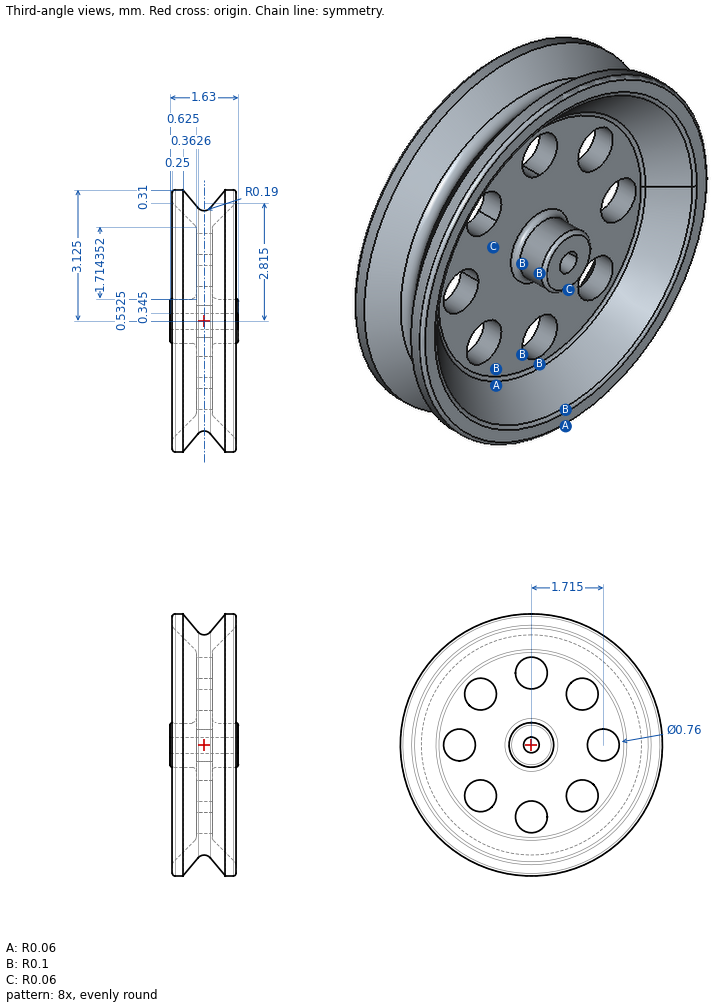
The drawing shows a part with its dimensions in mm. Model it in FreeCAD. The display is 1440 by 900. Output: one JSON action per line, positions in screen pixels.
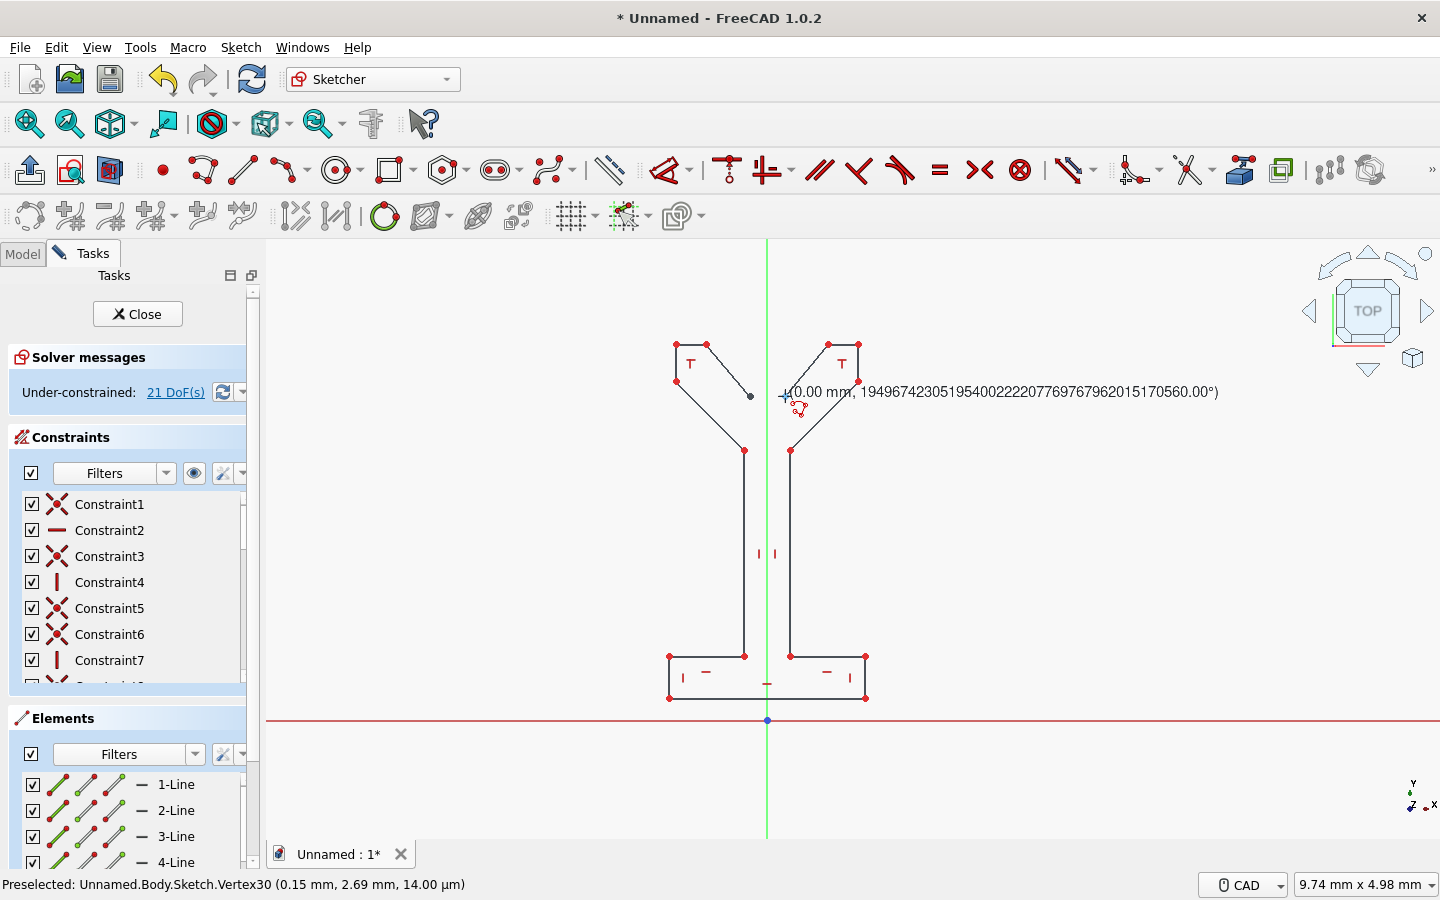
{"action": "left_click", "coordinate": [284, 170]}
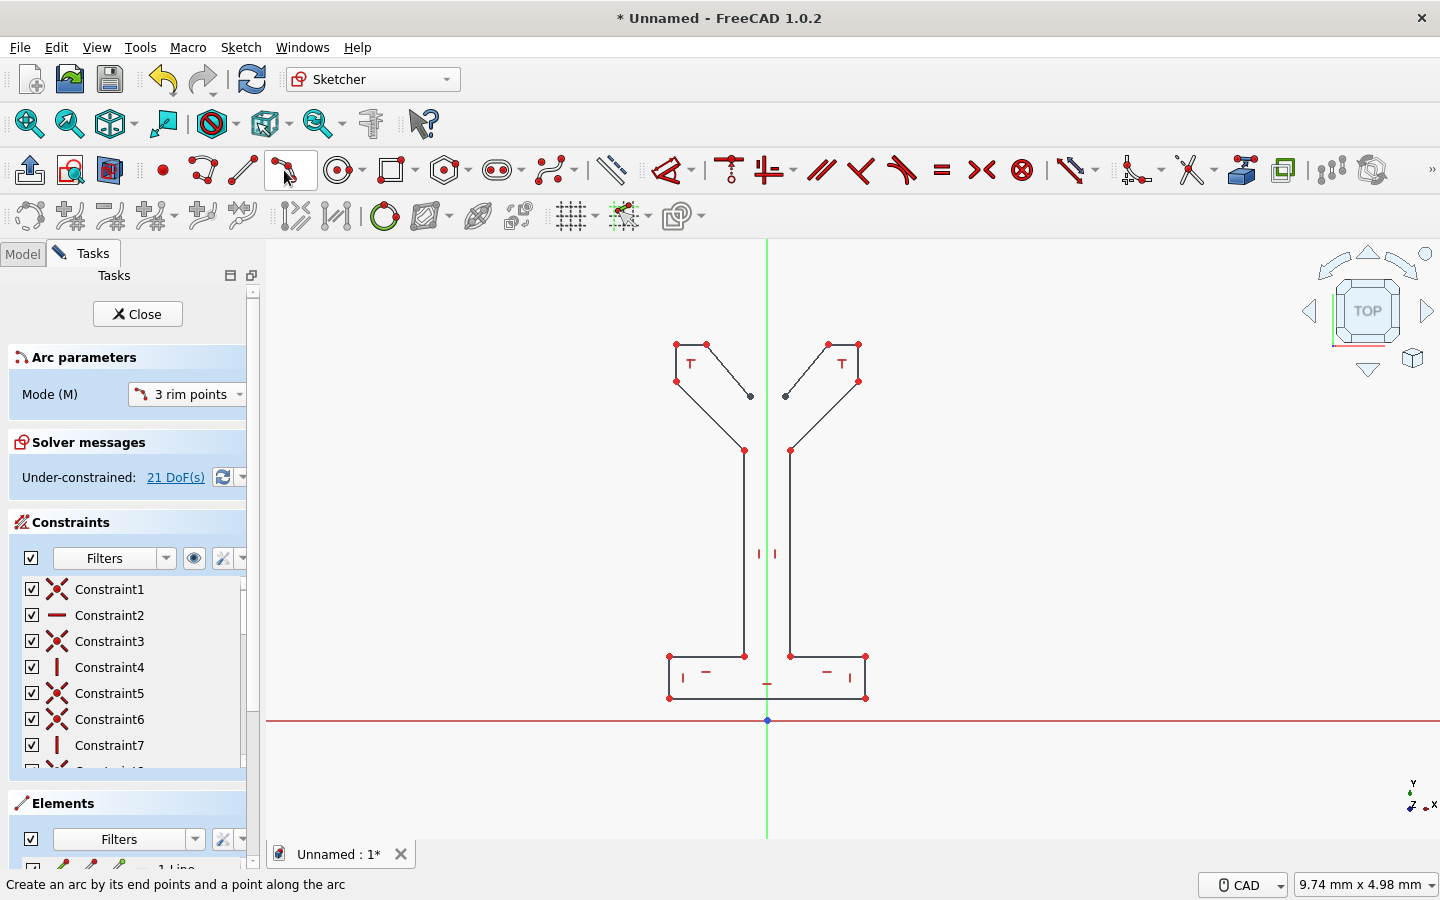
{"action": "left_click", "coordinate": [785, 397]}
{"action": "left_click", "coordinate": [750, 397]}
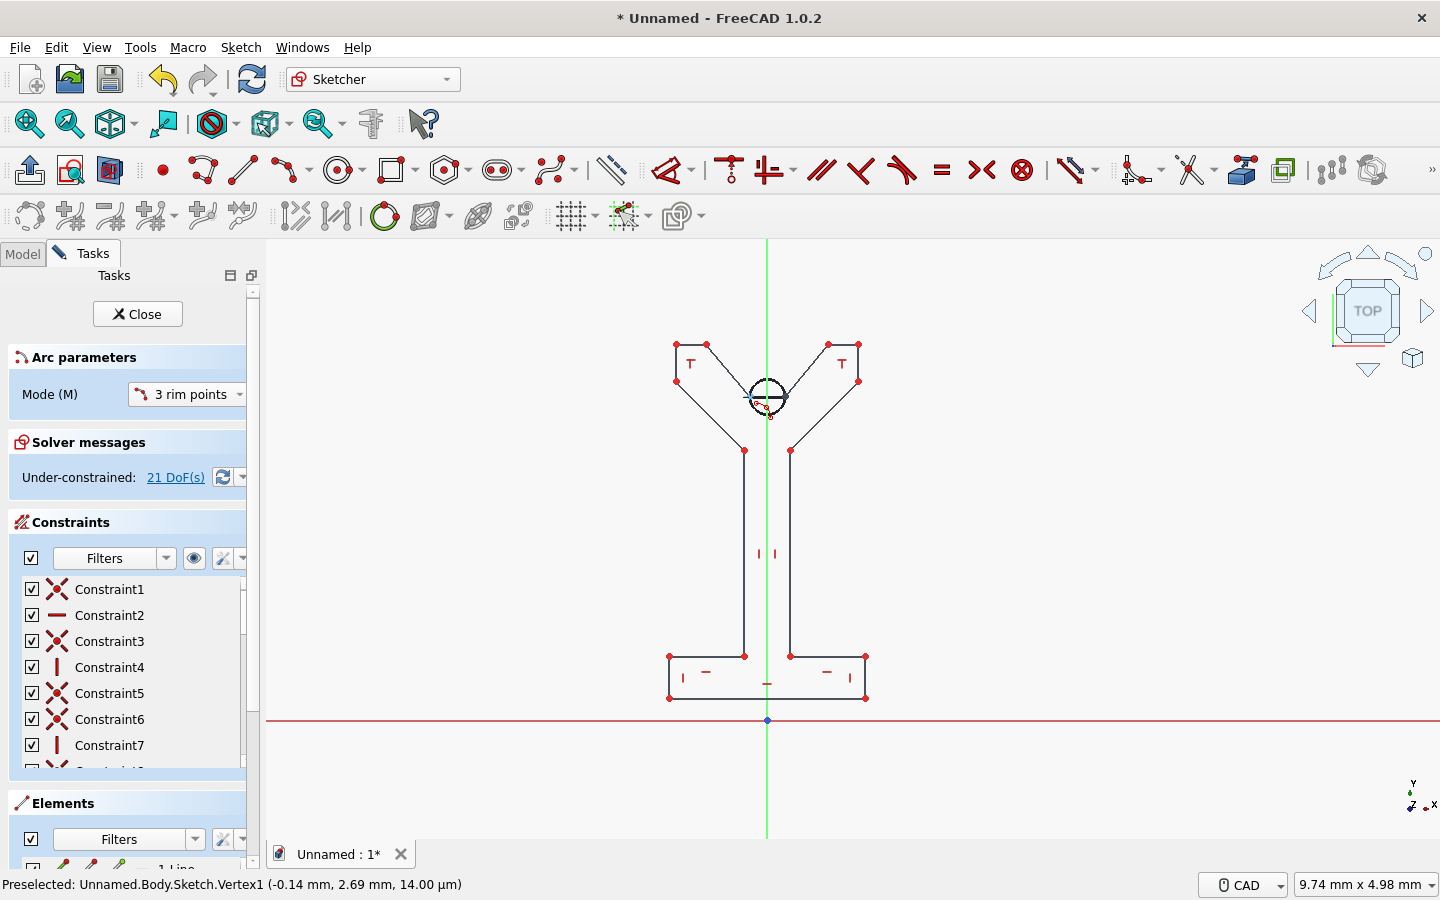
{"action": "scroll", "coordinate": [759, 403], "scroll_direction": "up", "scroll_amount": 5}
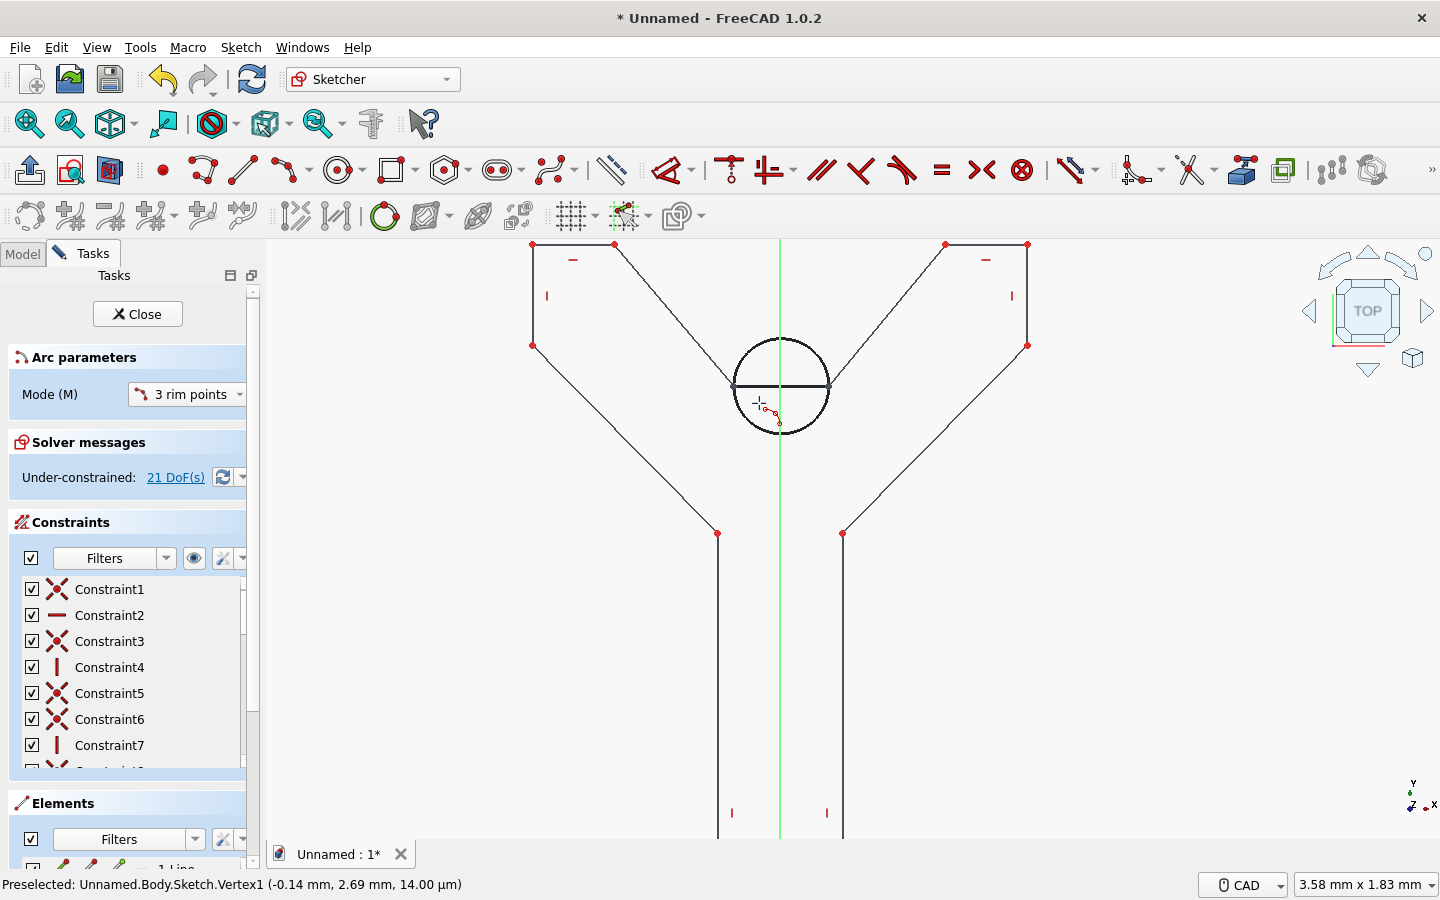
{"action": "left_click", "coordinate": [759, 402]}
{"action": "key", "text": "Escape"}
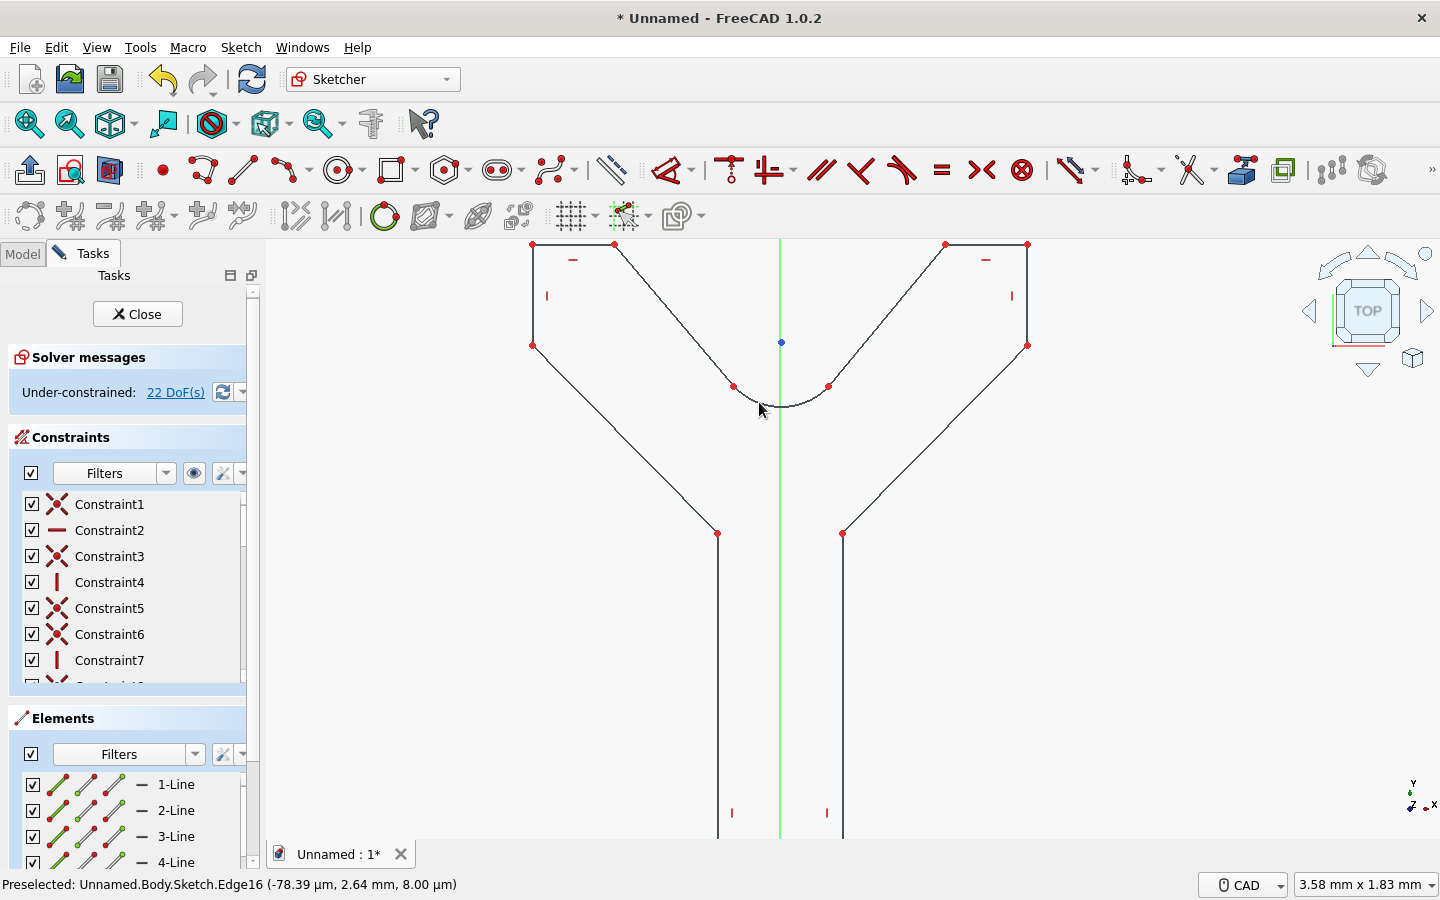
{"action": "left_click", "coordinate": [698, 344]}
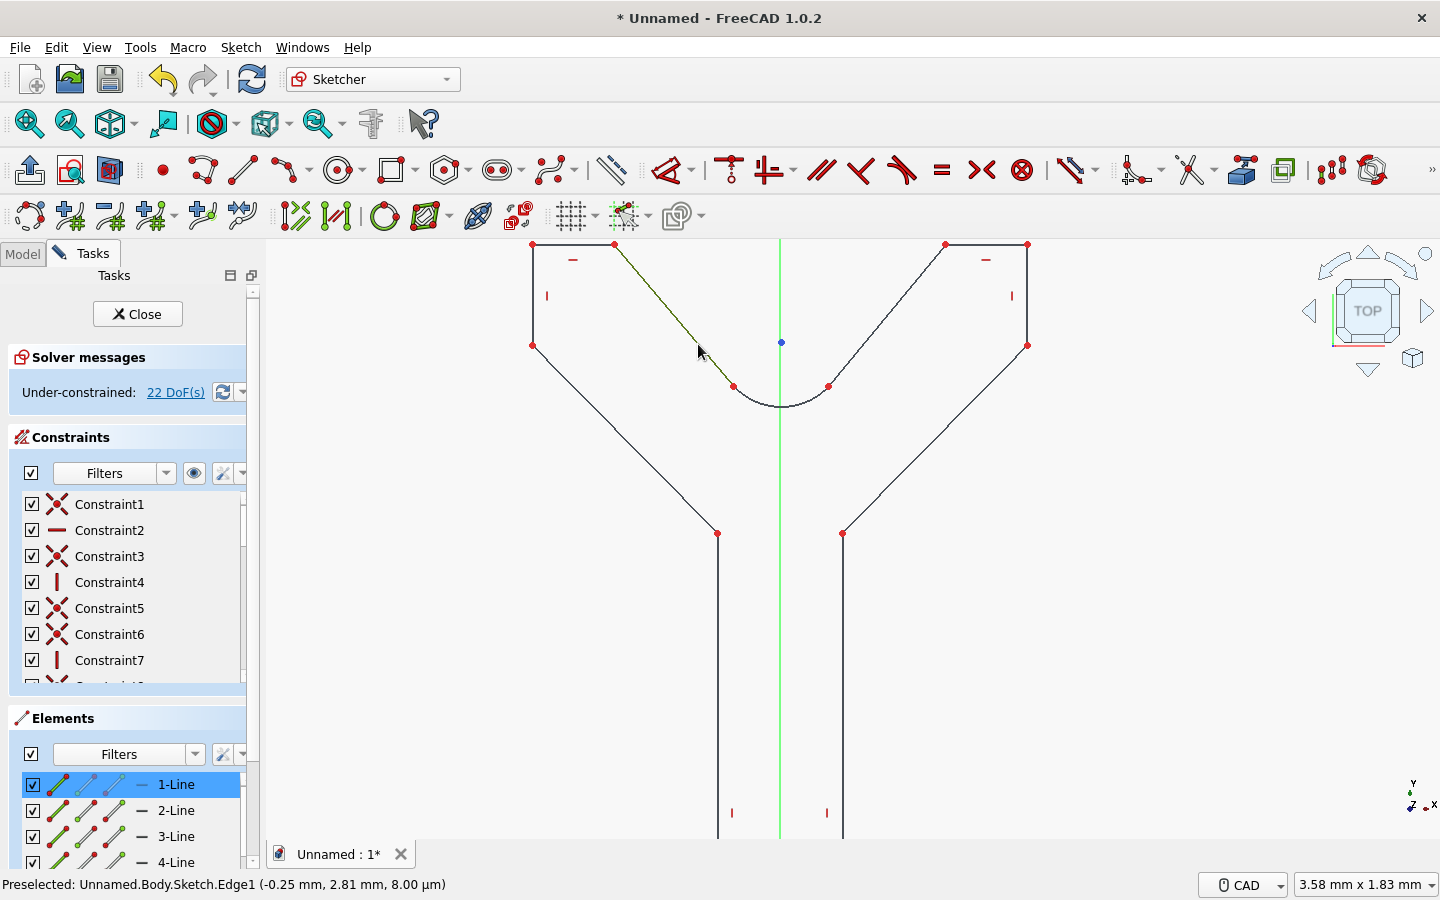
{"action": "left_click", "coordinate": [760, 403]}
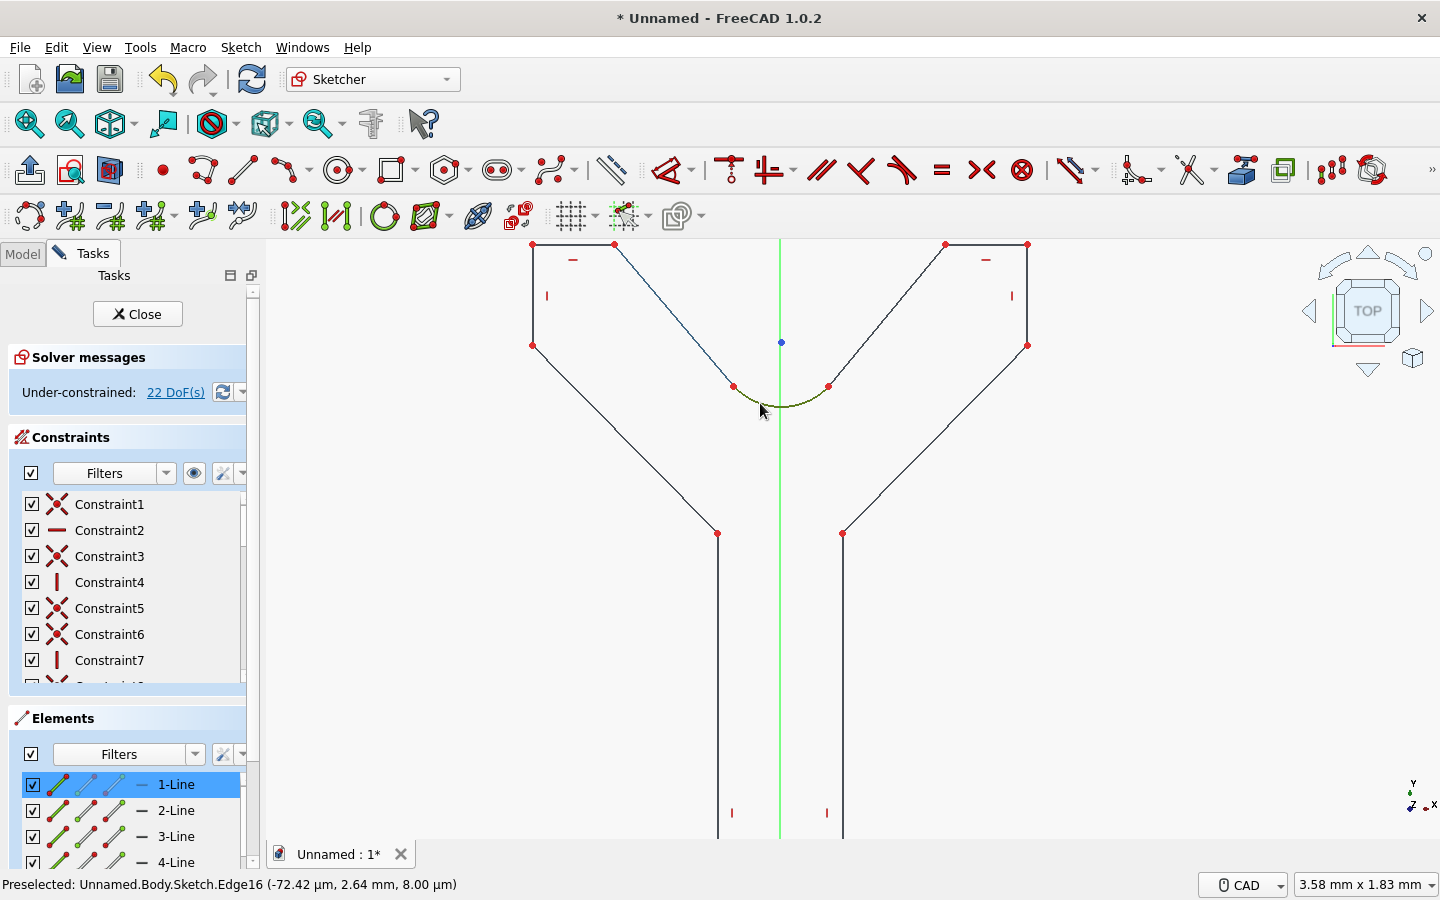
{"action": "key", "text": "t"}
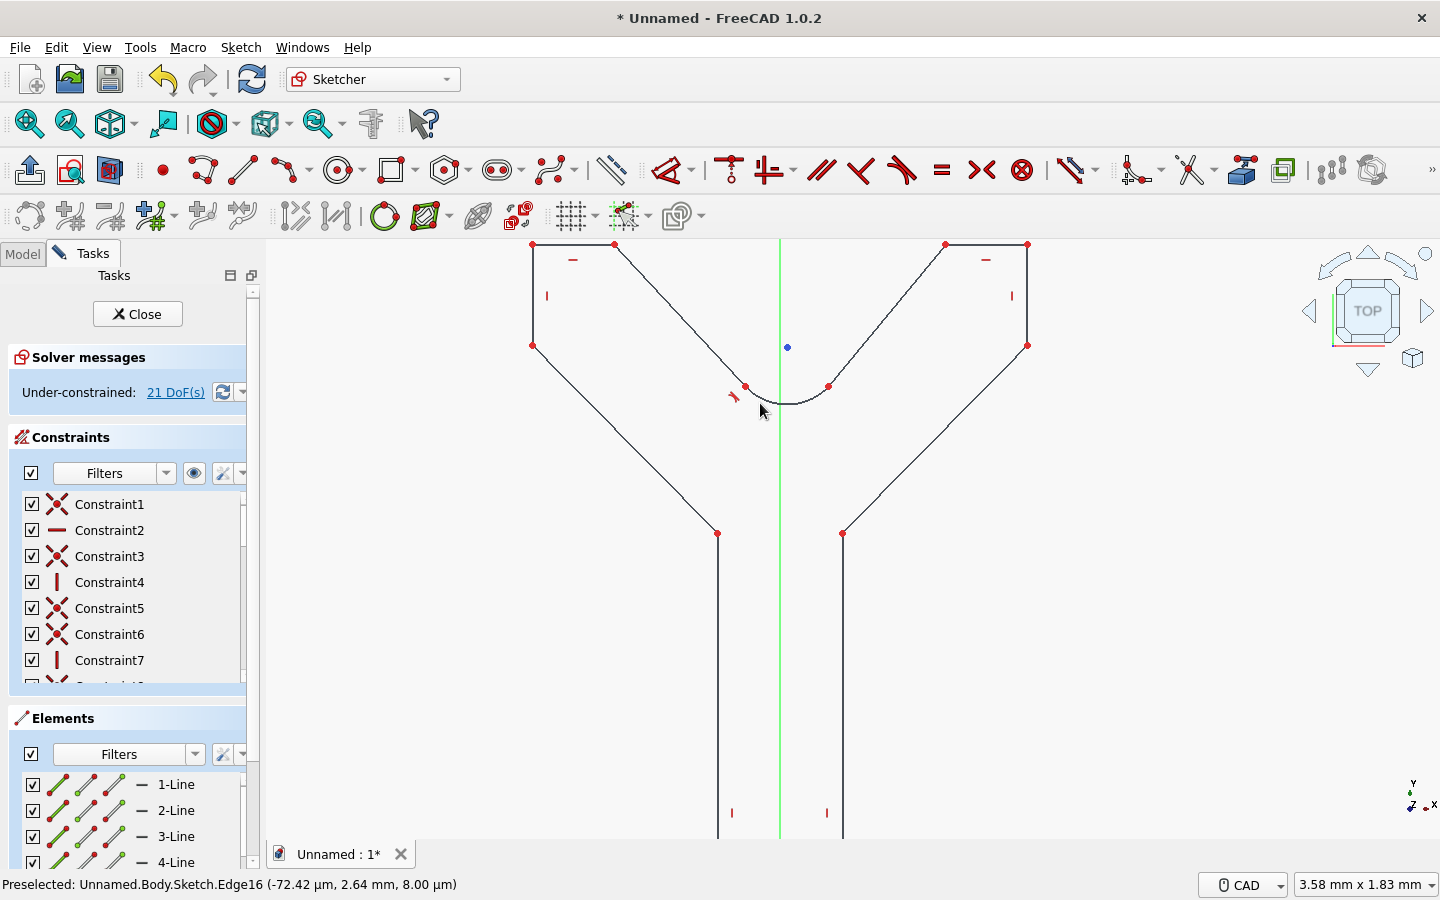
{"action": "left_click", "coordinate": [911, 287]}